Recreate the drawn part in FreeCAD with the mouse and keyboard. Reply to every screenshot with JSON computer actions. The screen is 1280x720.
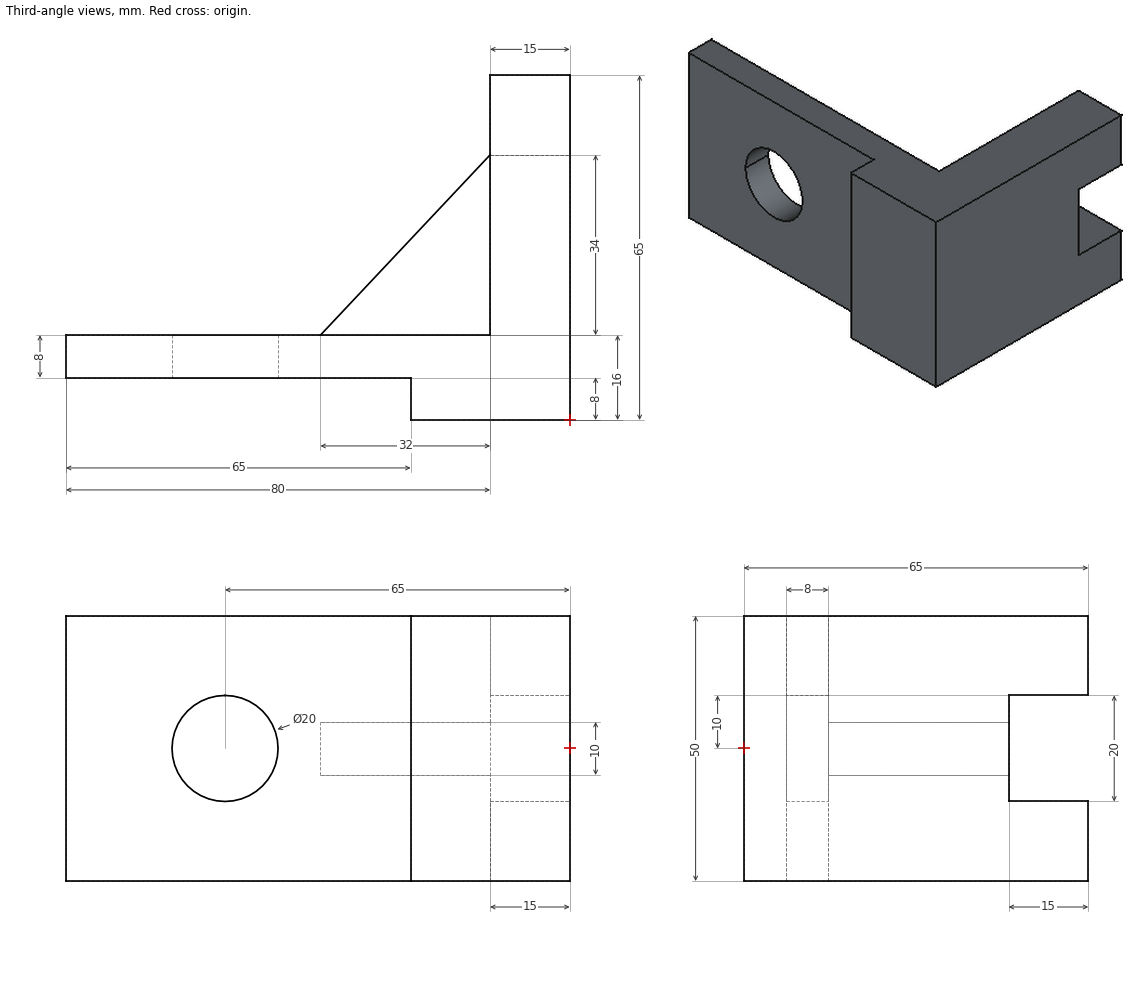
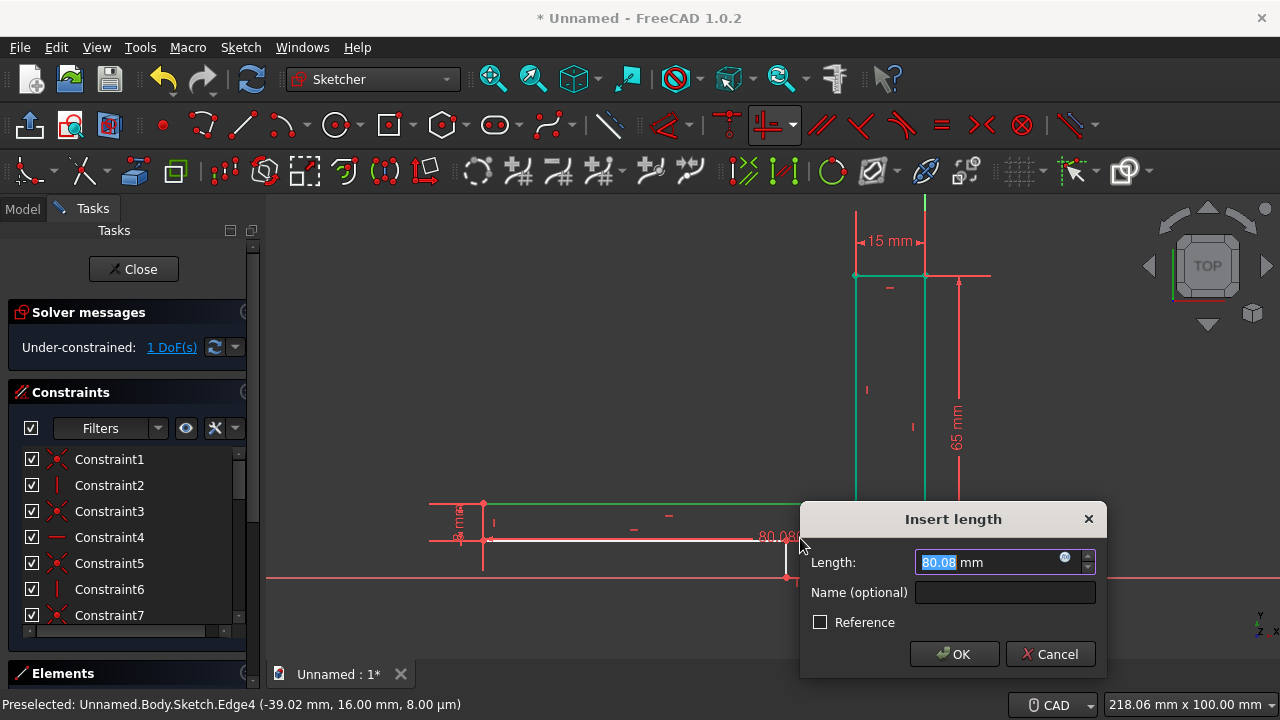
{"action": "type", "text": "80"}
{"action": "key", "text": "Return"}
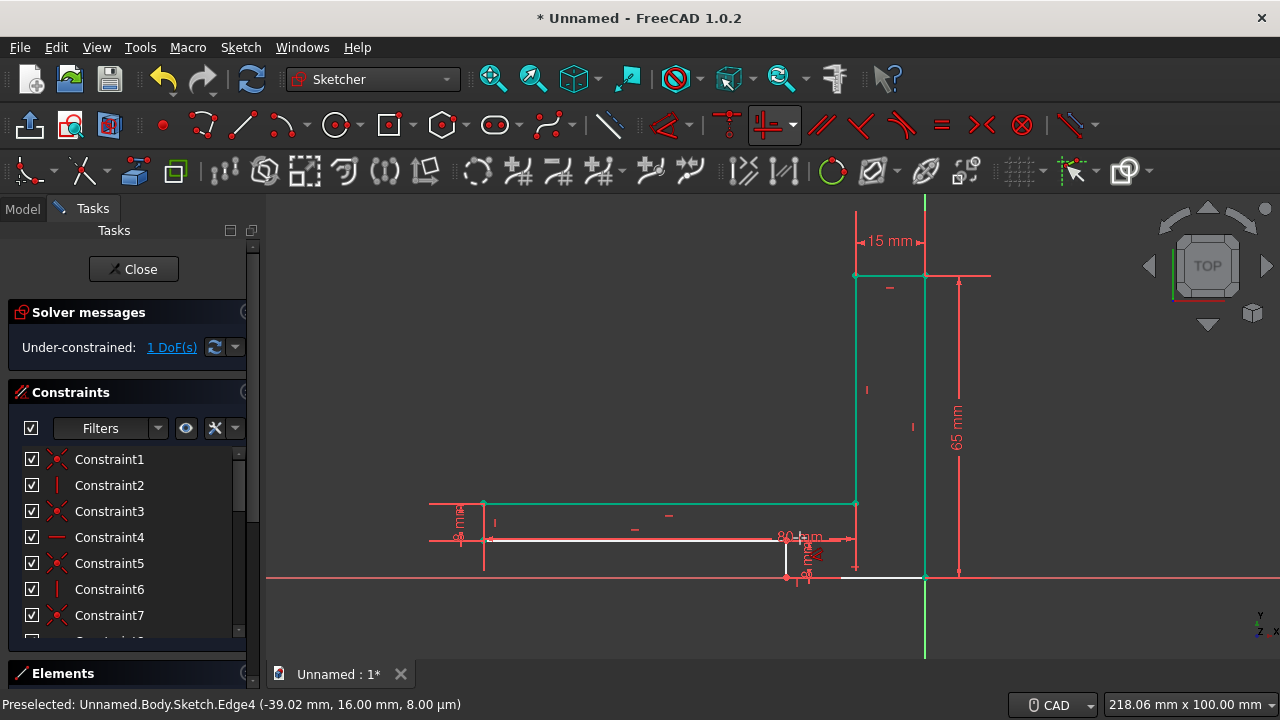
{"action": "left_click", "coordinate": [574, 541]}
{"action": "left_click", "coordinate": [635, 599]}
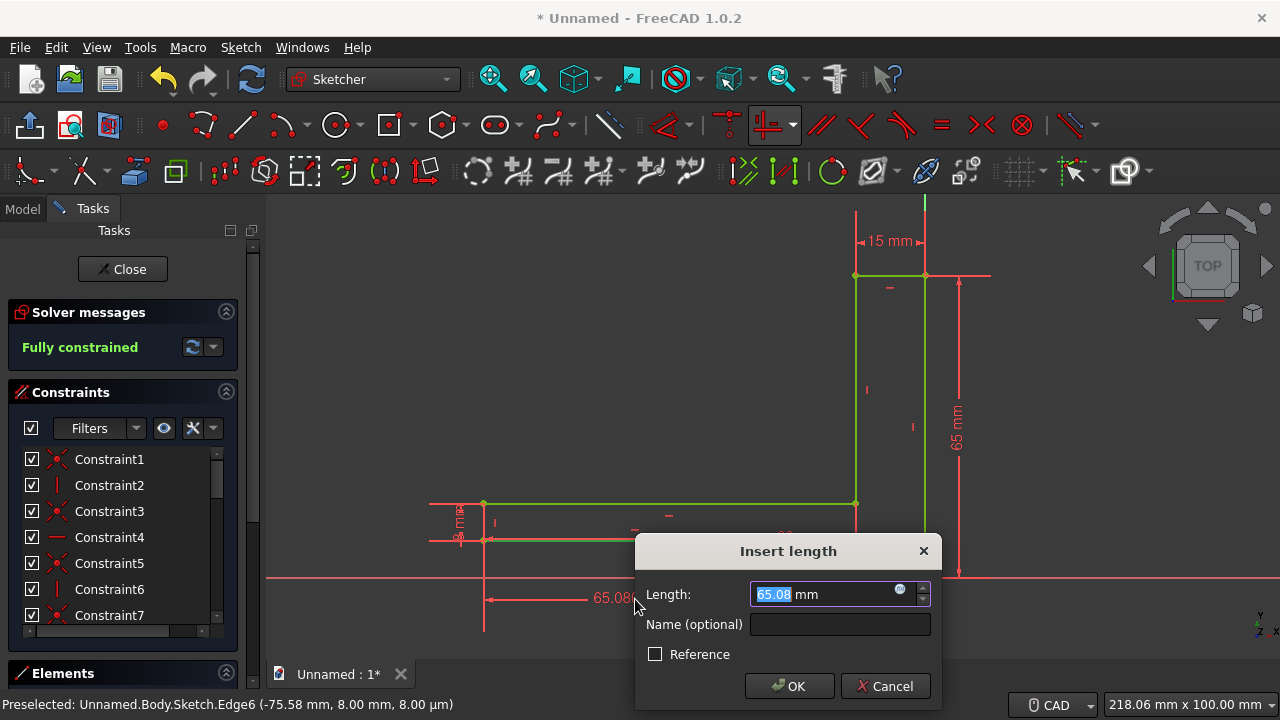
{"action": "type", "text": "65"}
{"action": "key", "text": "Return"}
{"action": "key", "text": "Escape"}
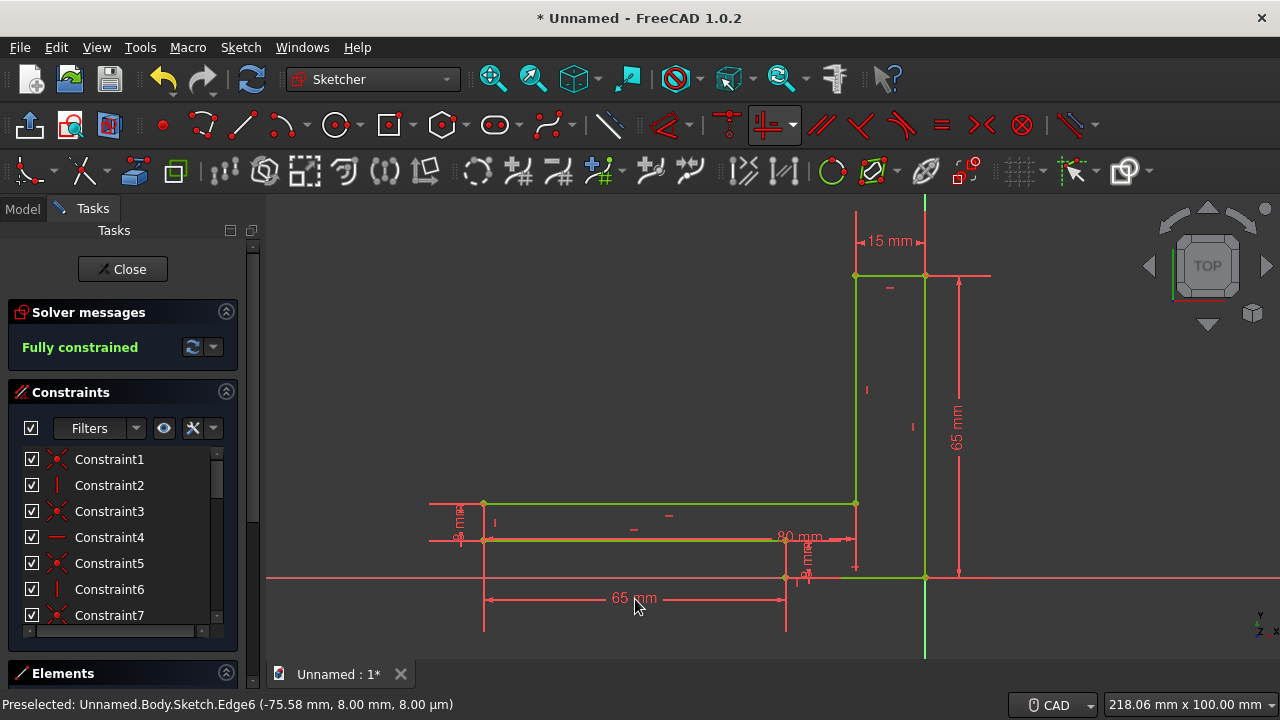
{"action": "left_click", "coordinate": [123, 269]}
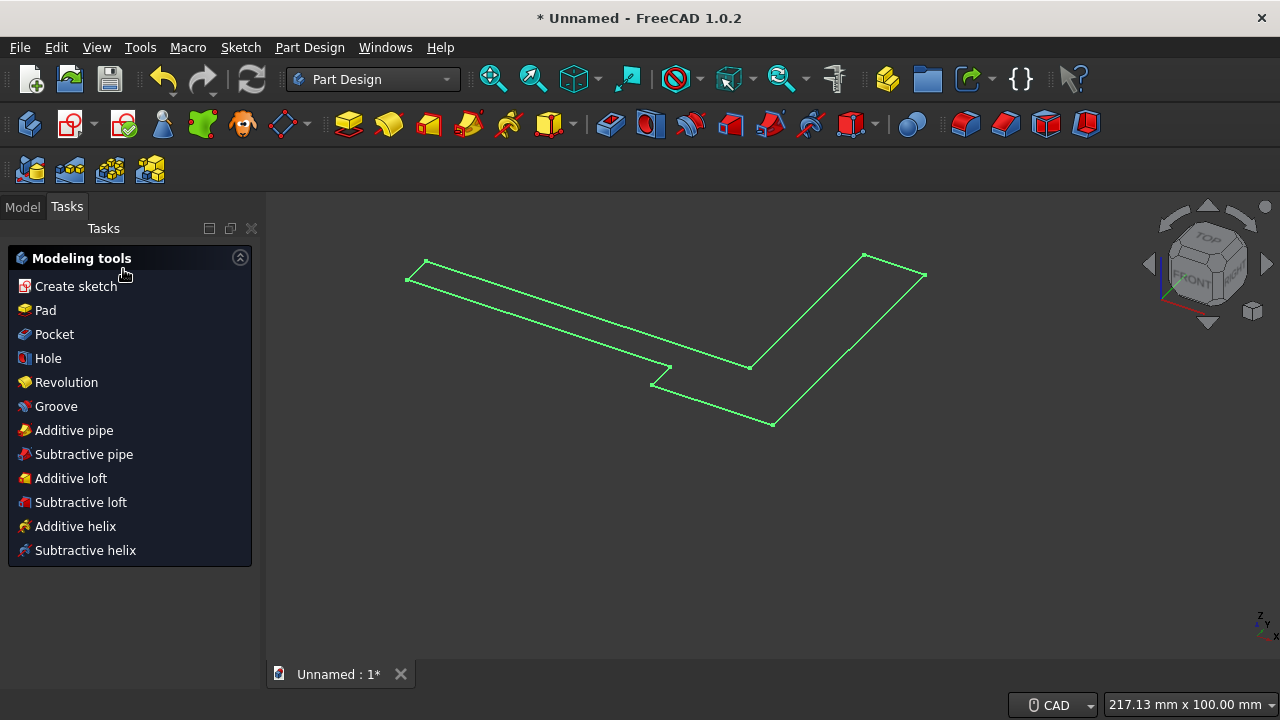
{"action": "left_click", "coordinate": [350, 124]}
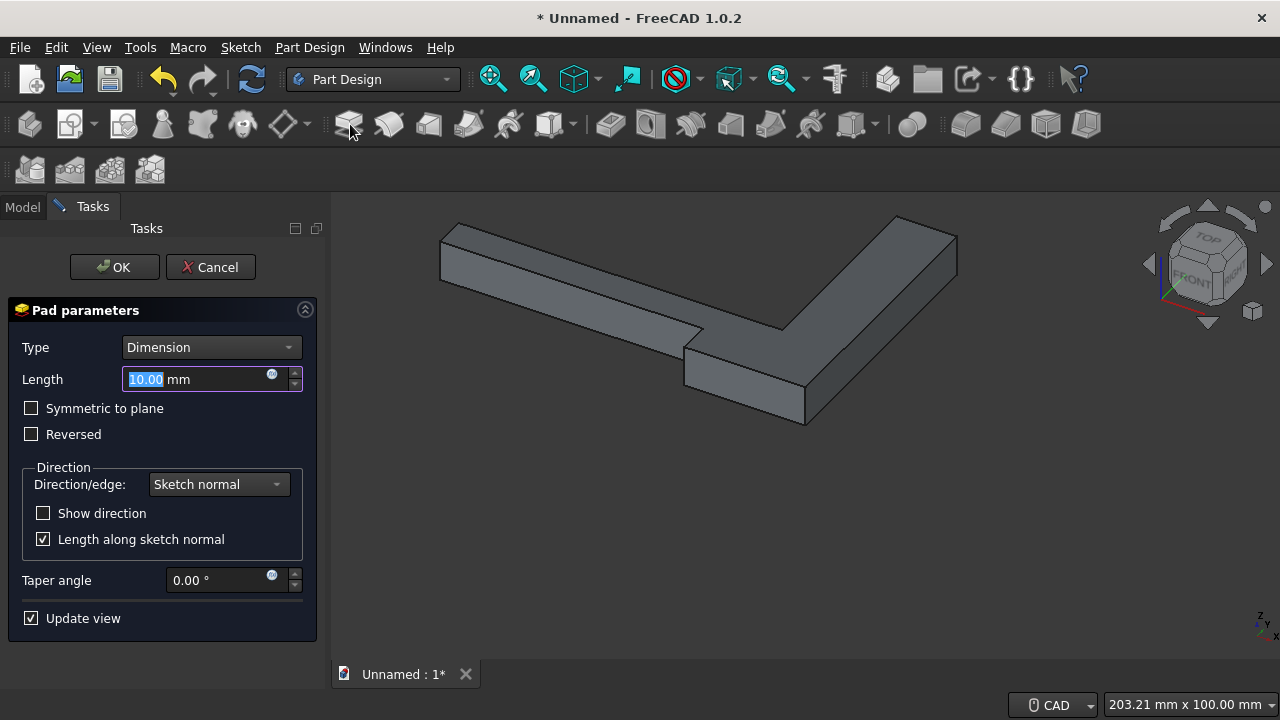
{"action": "type", "text": "50"}
{"action": "key", "text": "Tab"}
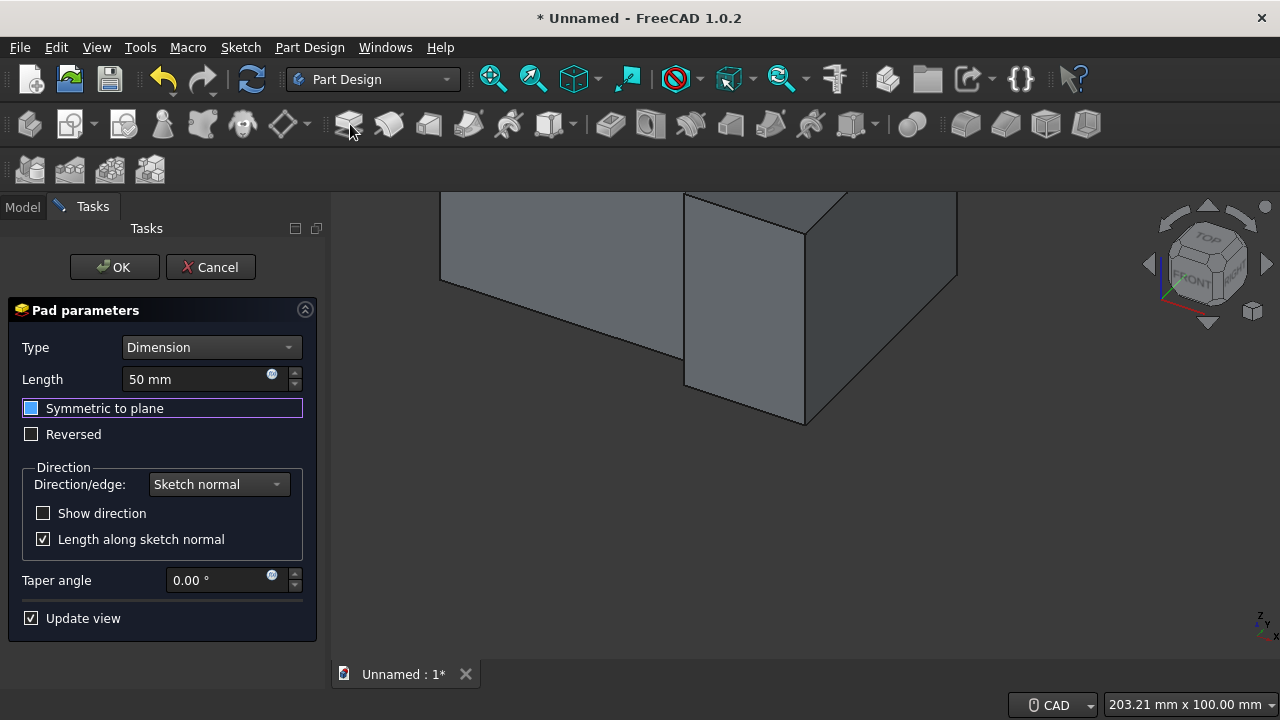
{"action": "left_click", "coordinate": [30, 408]}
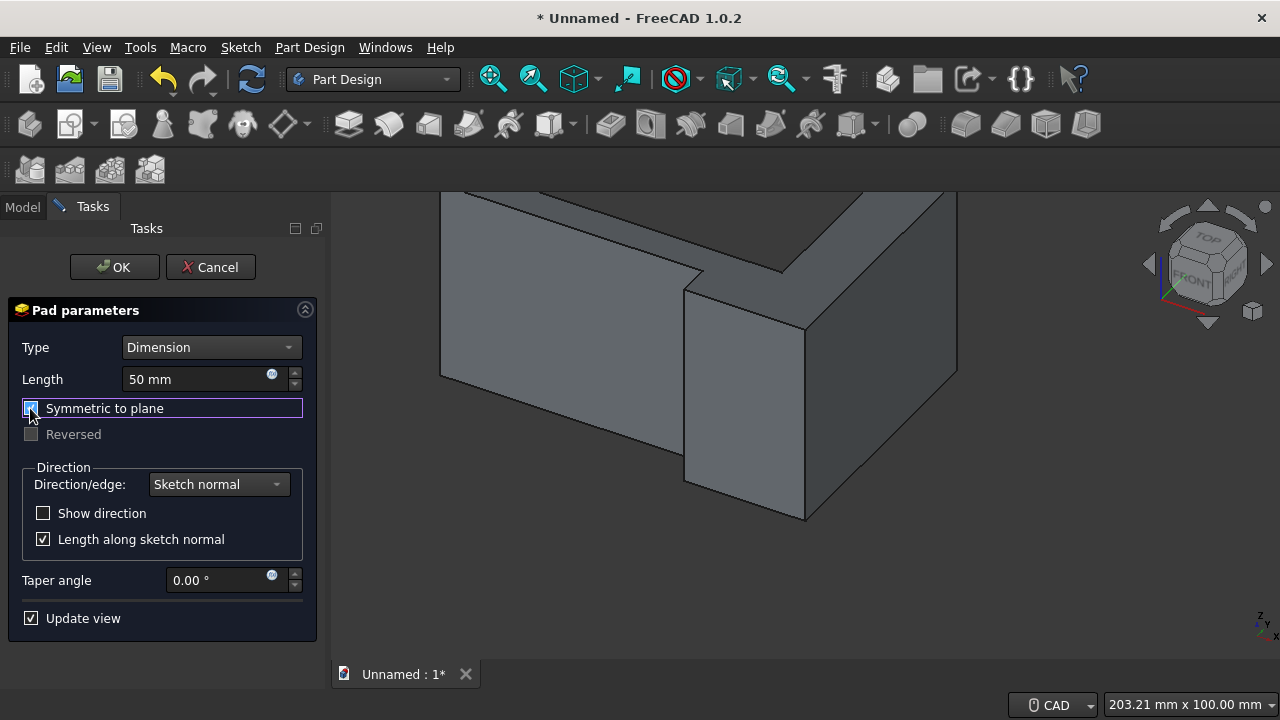
{"action": "left_click", "coordinate": [115, 267]}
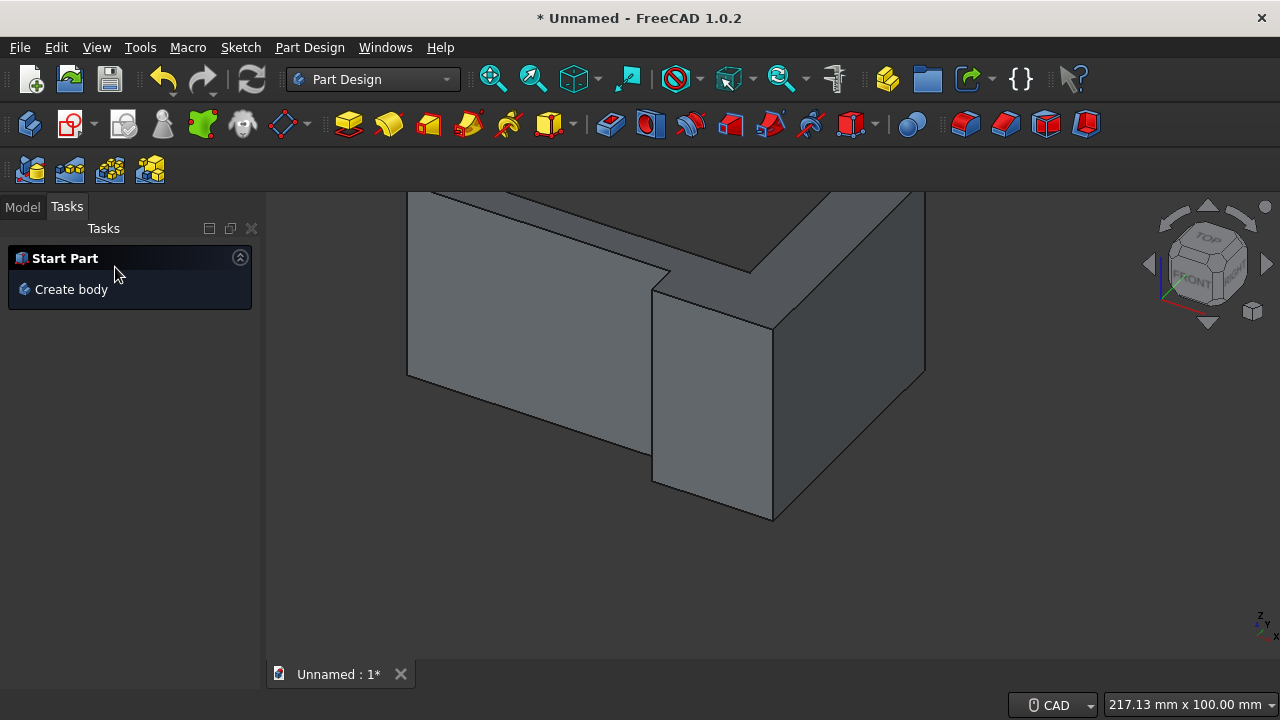
{"action": "key", "text": "v f"}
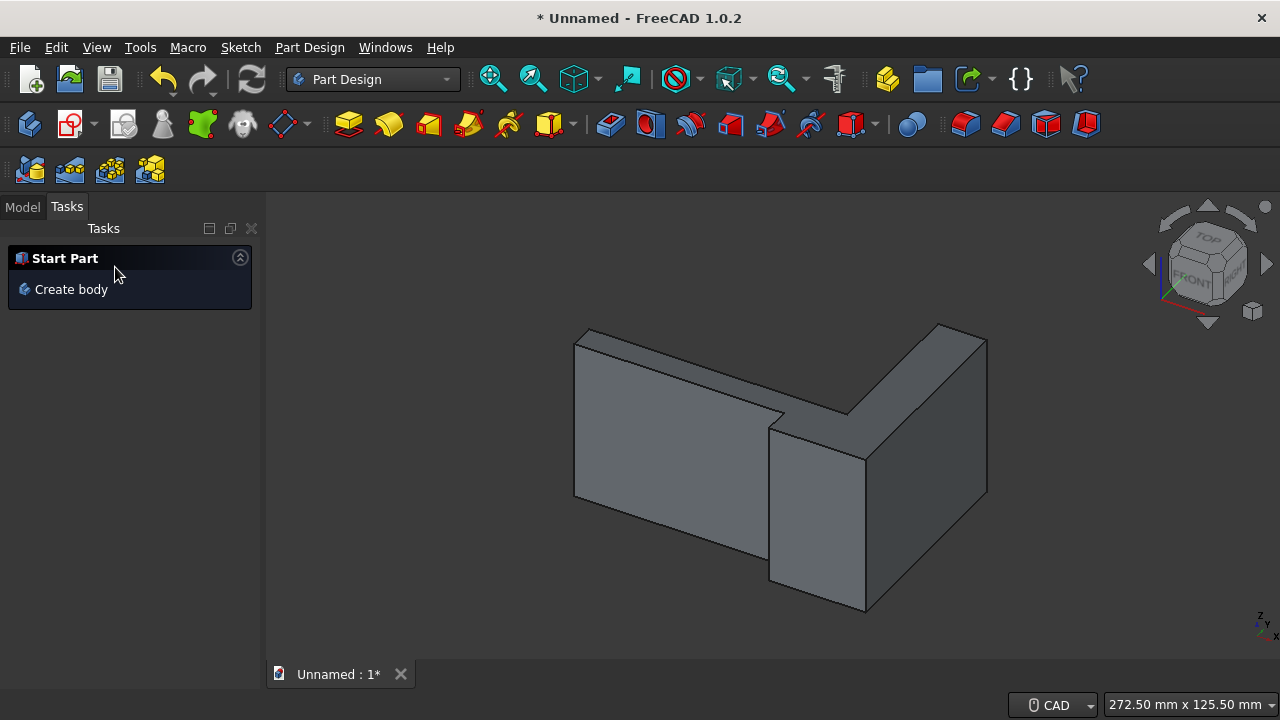
{"action": "key", "text": "6"}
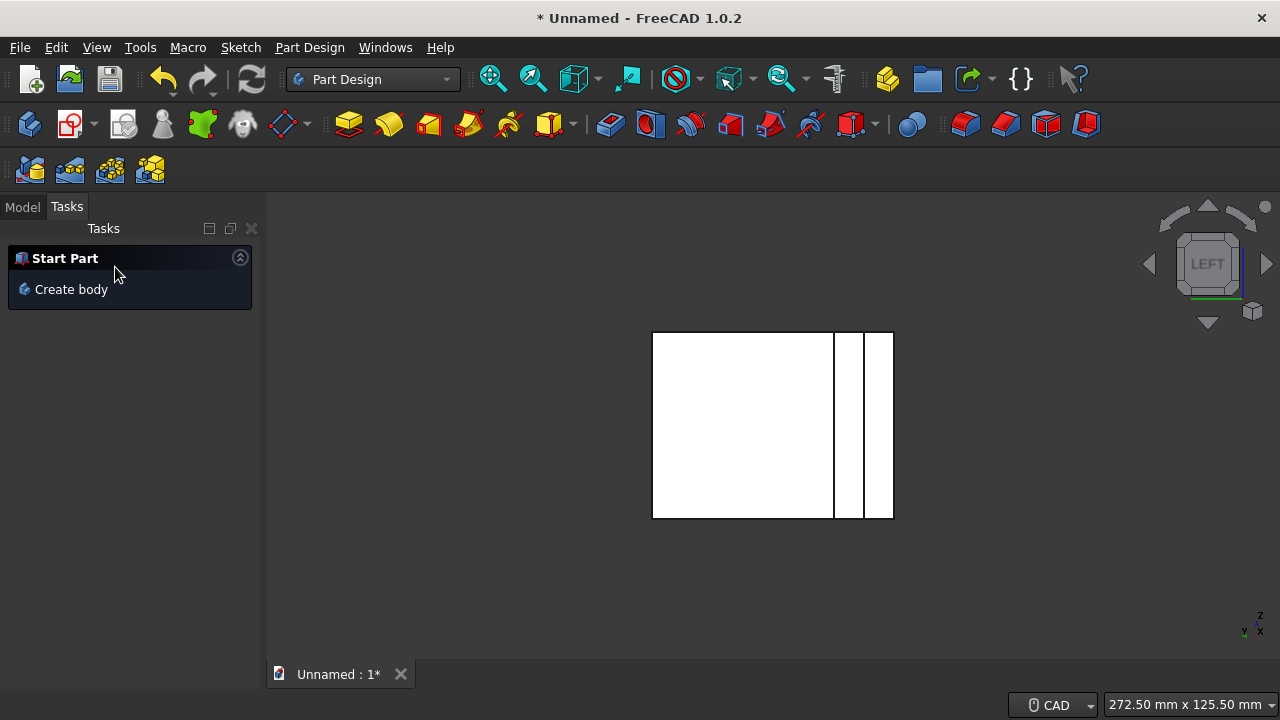
{"action": "key", "text": "v f"}